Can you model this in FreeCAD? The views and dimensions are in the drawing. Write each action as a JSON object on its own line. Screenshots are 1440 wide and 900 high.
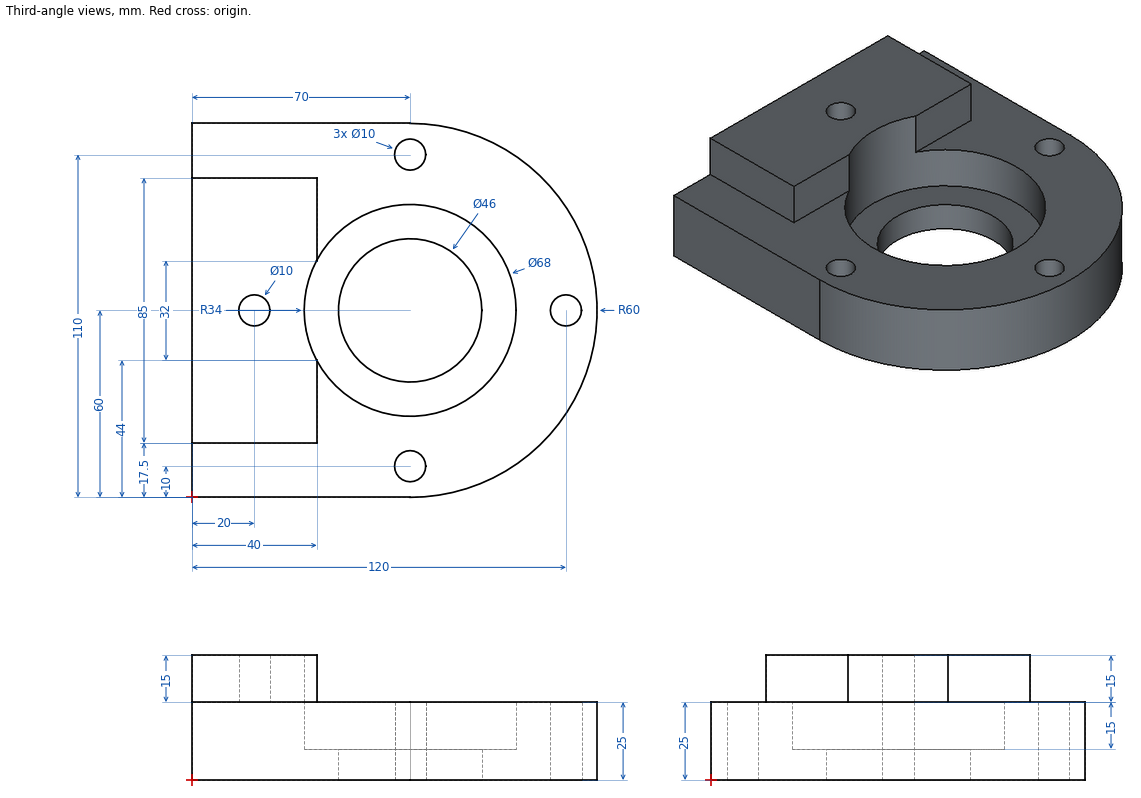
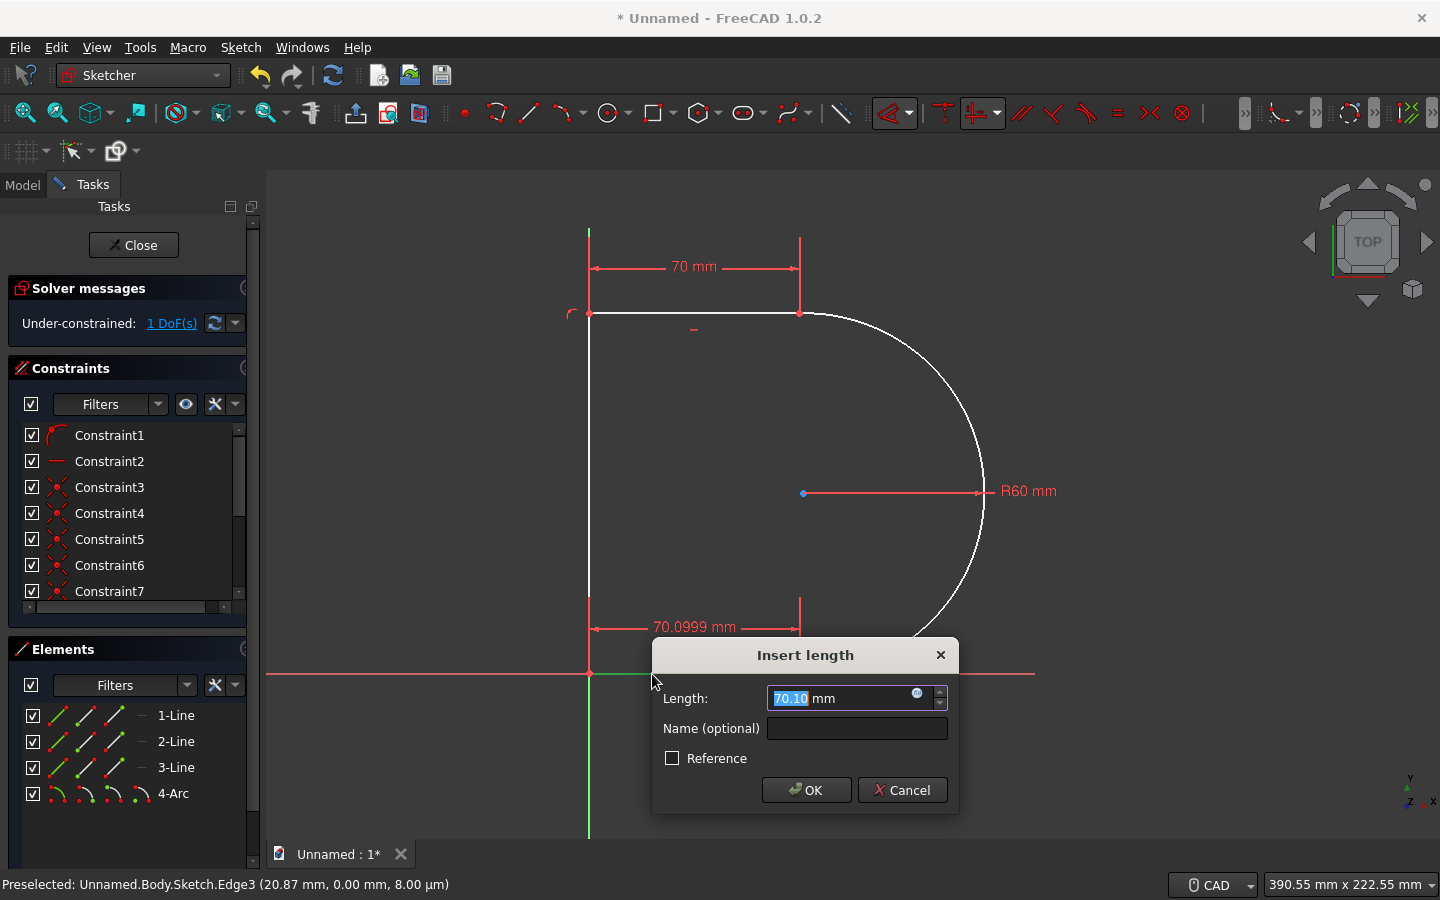
{"action": "type", "text": "70"}
{"action": "key", "text": "Return"}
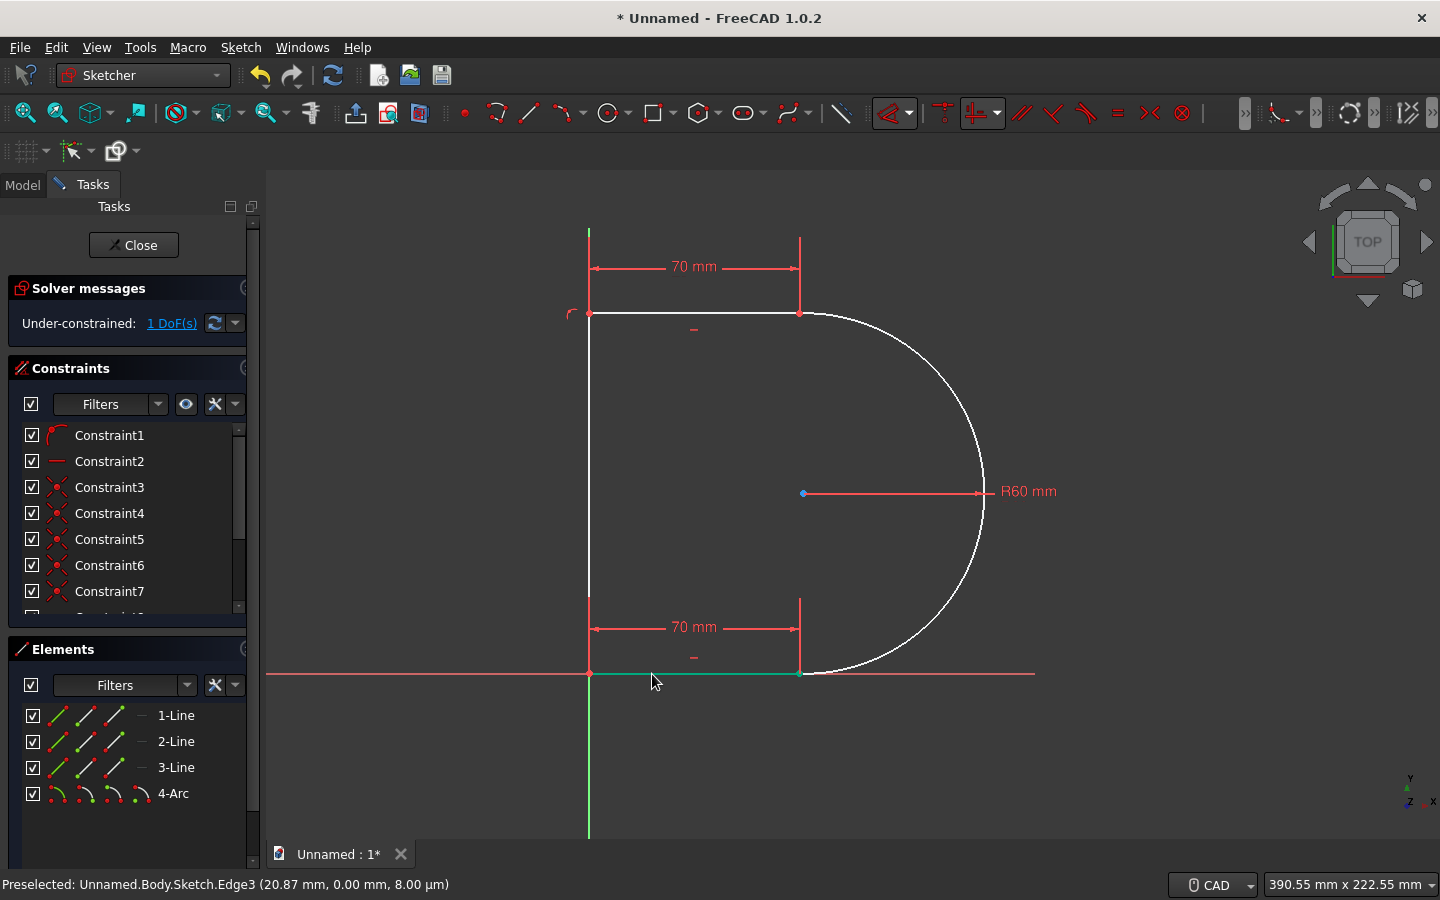
{"action": "left_click", "coordinate": [804, 493]}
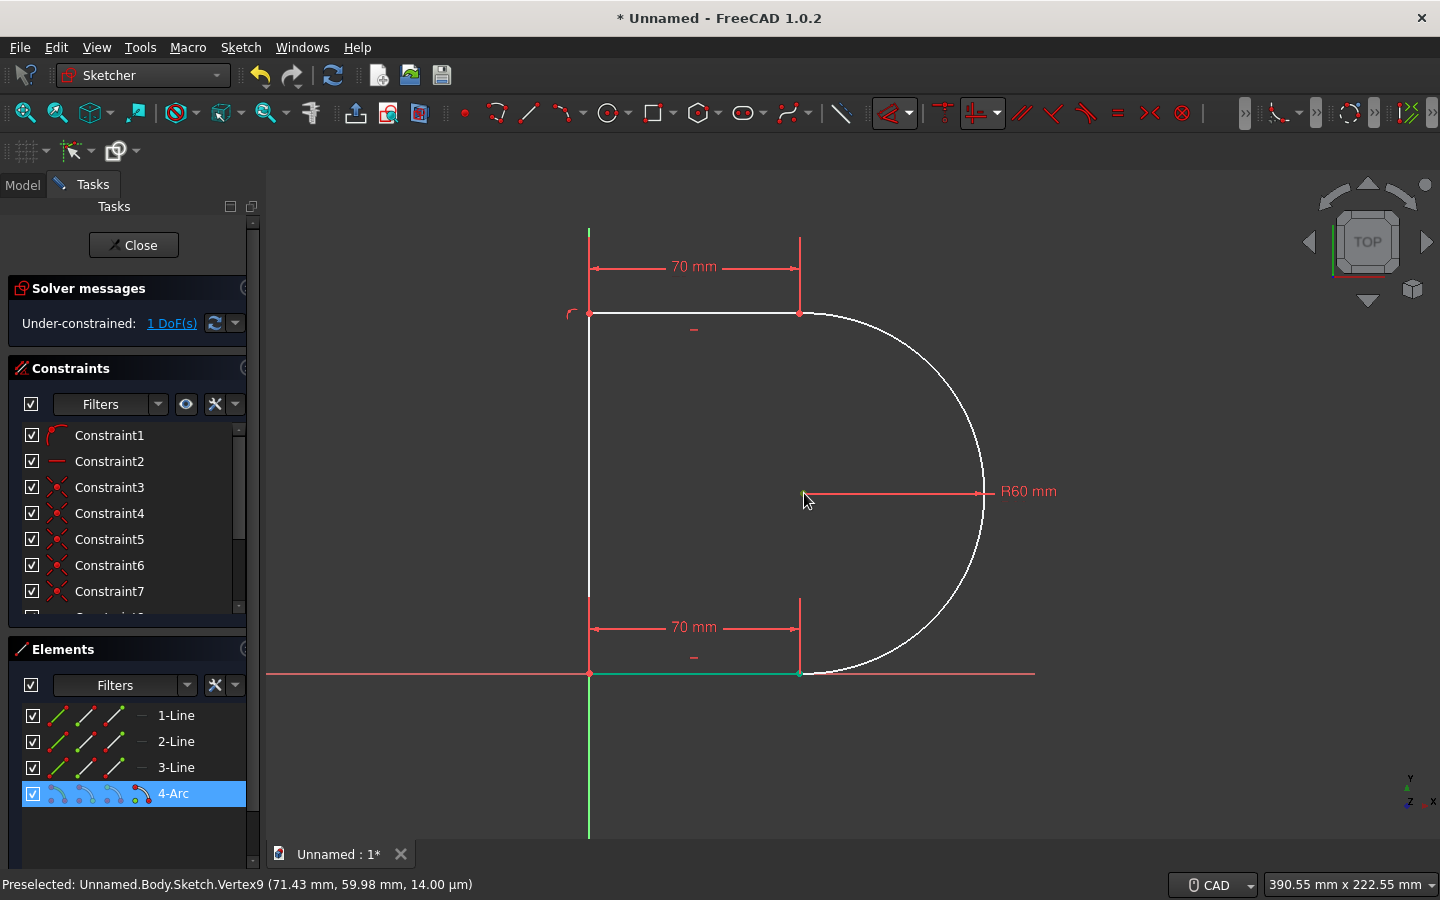
{"action": "left_click", "coordinate": [912, 114]}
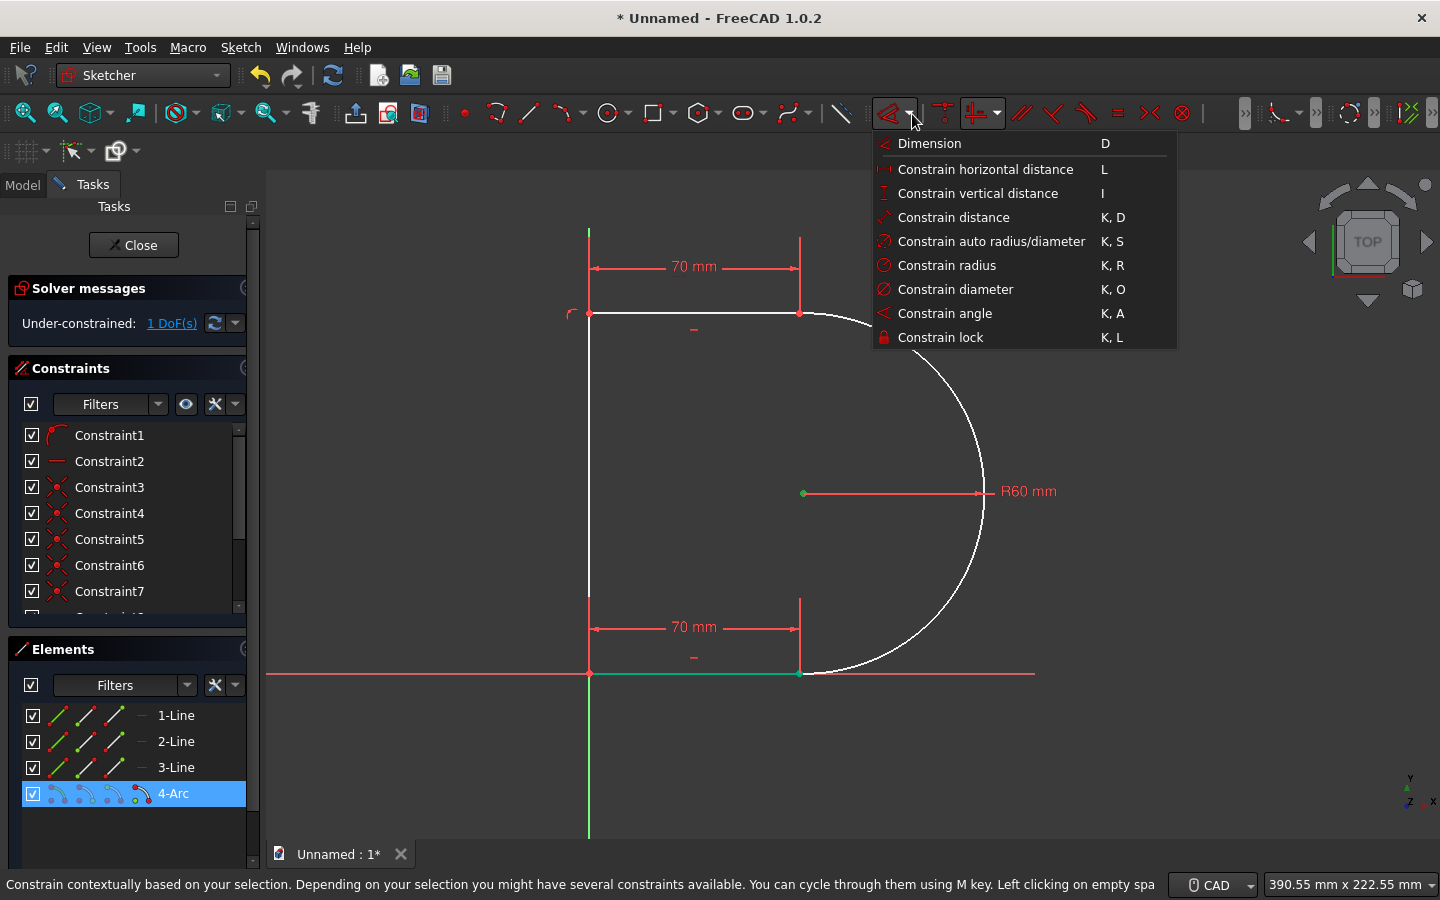
{"action": "left_click", "coordinate": [1025, 169]}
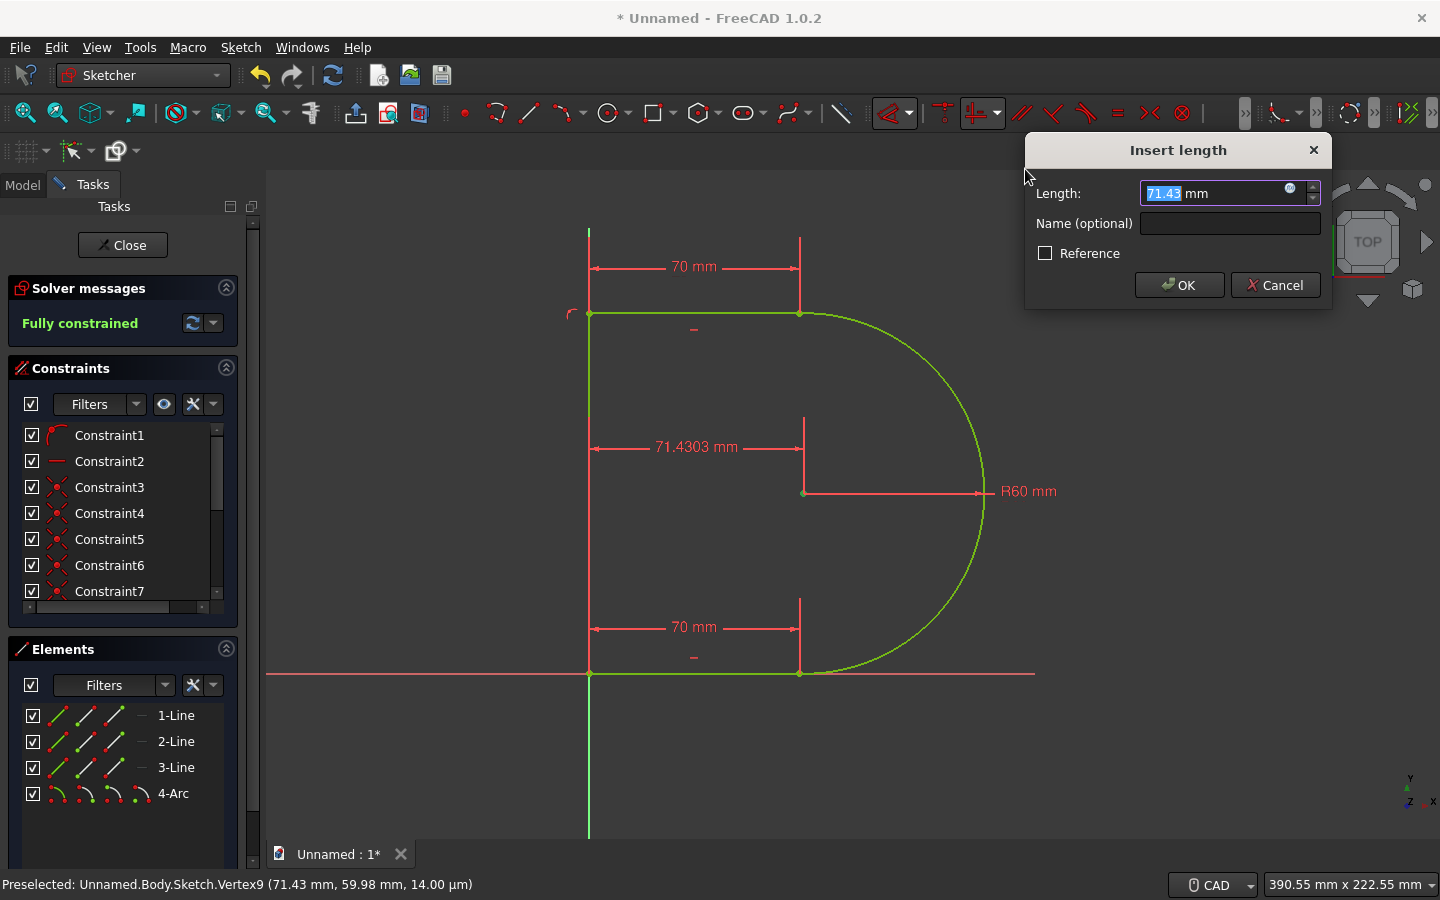
{"action": "type", "text": "70"}
{"action": "key", "text": "Return"}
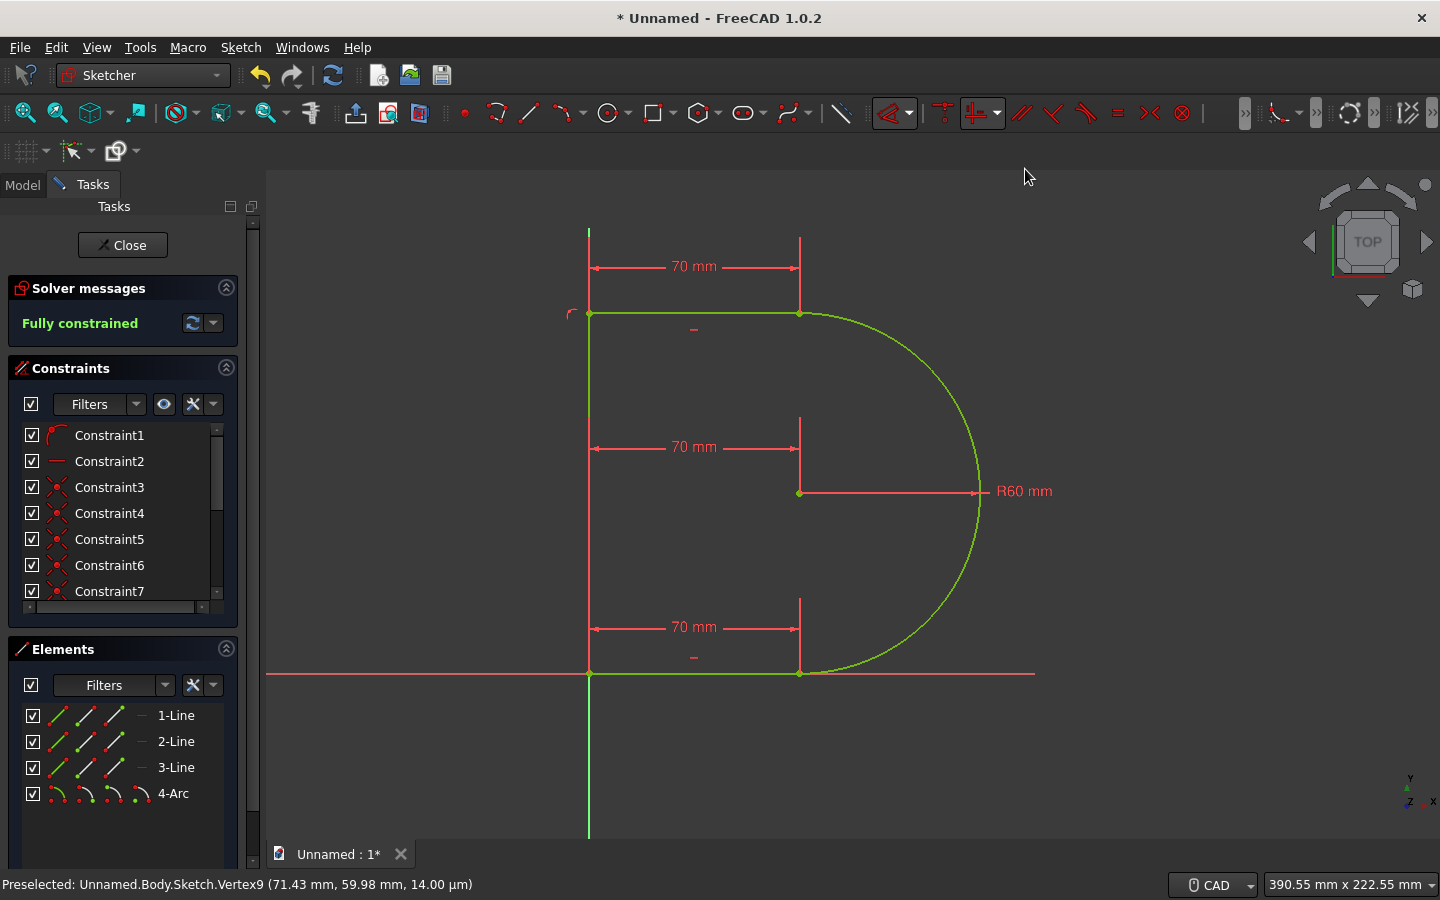
{"action": "left_click", "coordinate": [123, 245]}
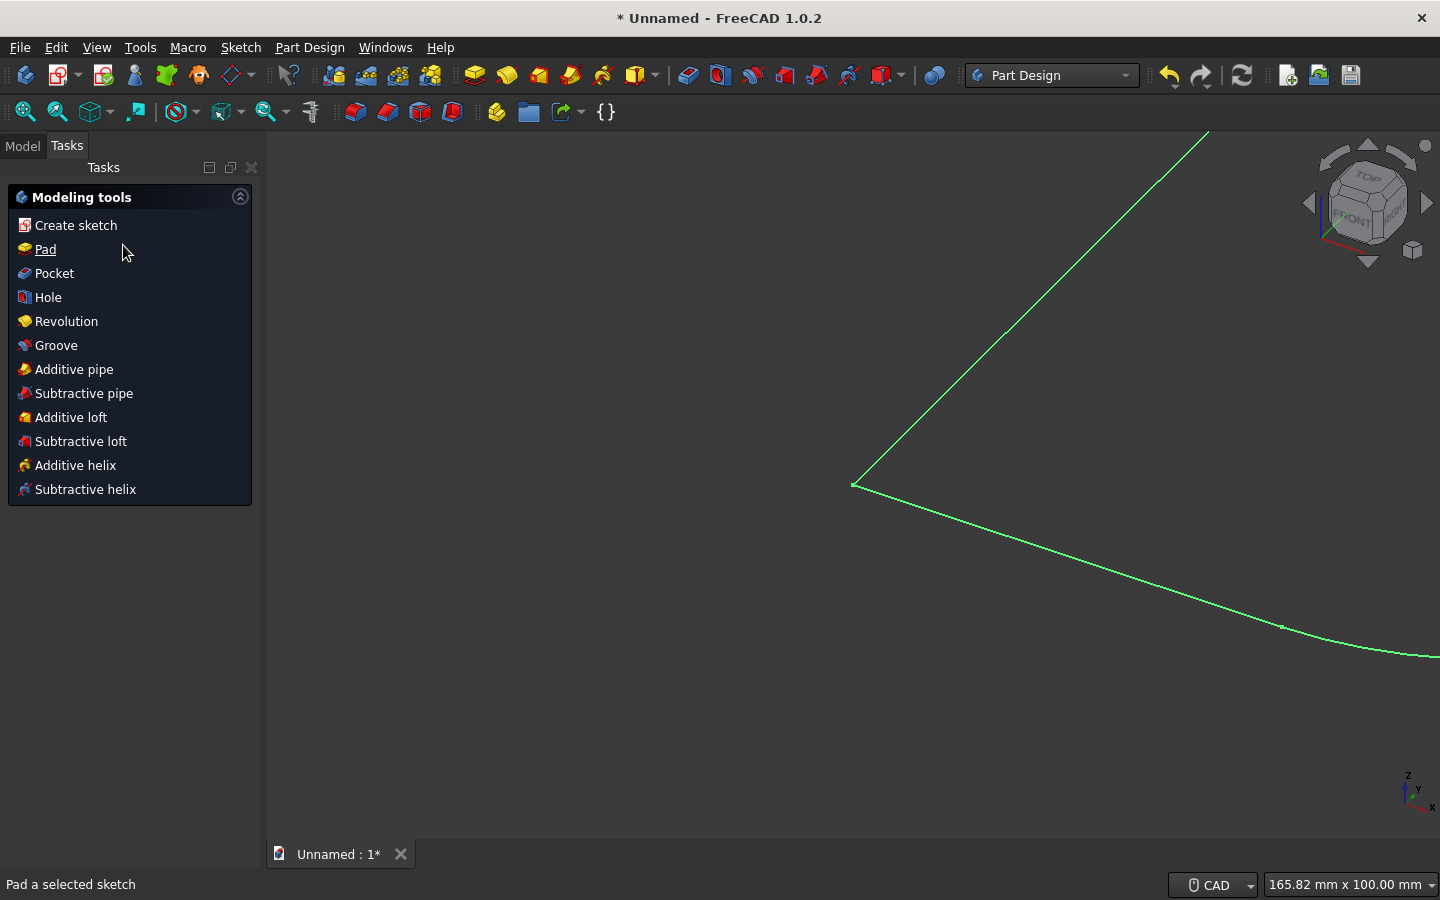
{"action": "left_click", "coordinate": [476, 76]}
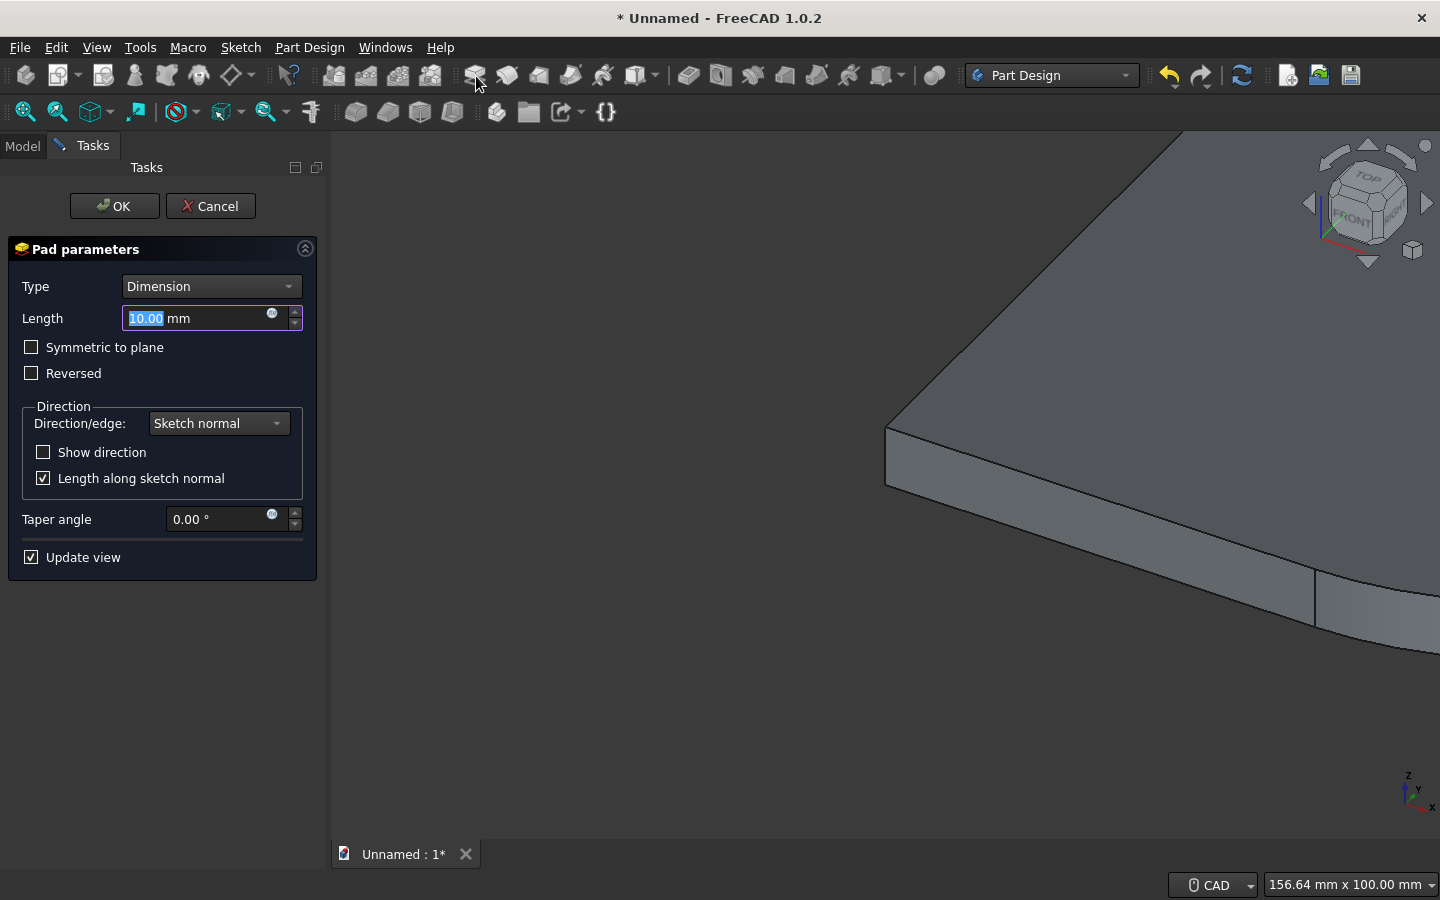
{"action": "type", "text": "25"}
{"action": "key", "text": "Tab"}